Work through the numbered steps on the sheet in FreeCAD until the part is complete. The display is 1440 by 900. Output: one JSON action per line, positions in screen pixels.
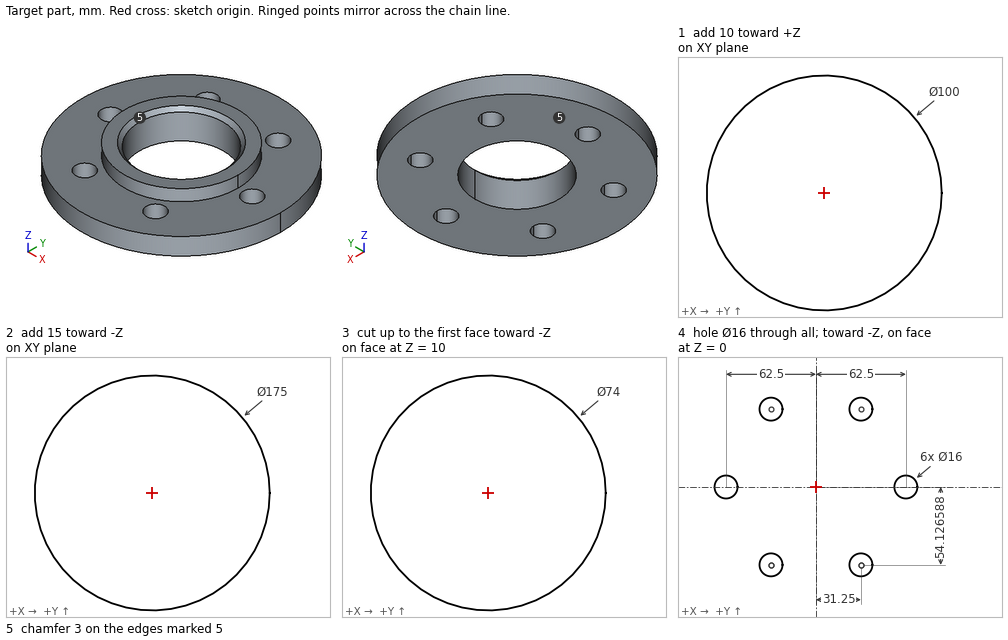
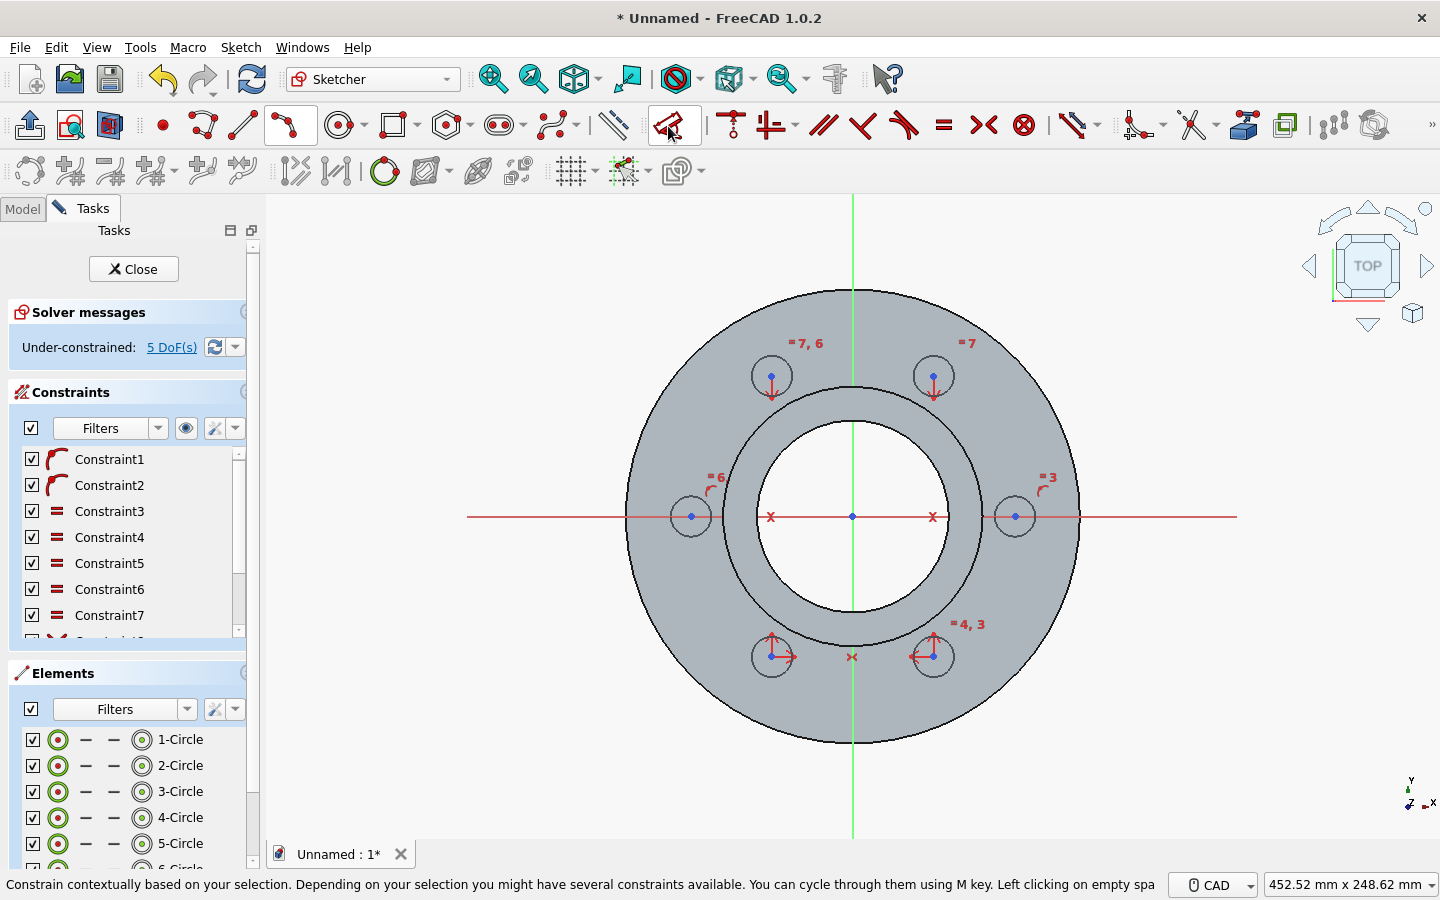
{"action": "left_click", "coordinate": [1029, 502]}
{"action": "left_click", "coordinate": [1051, 479]}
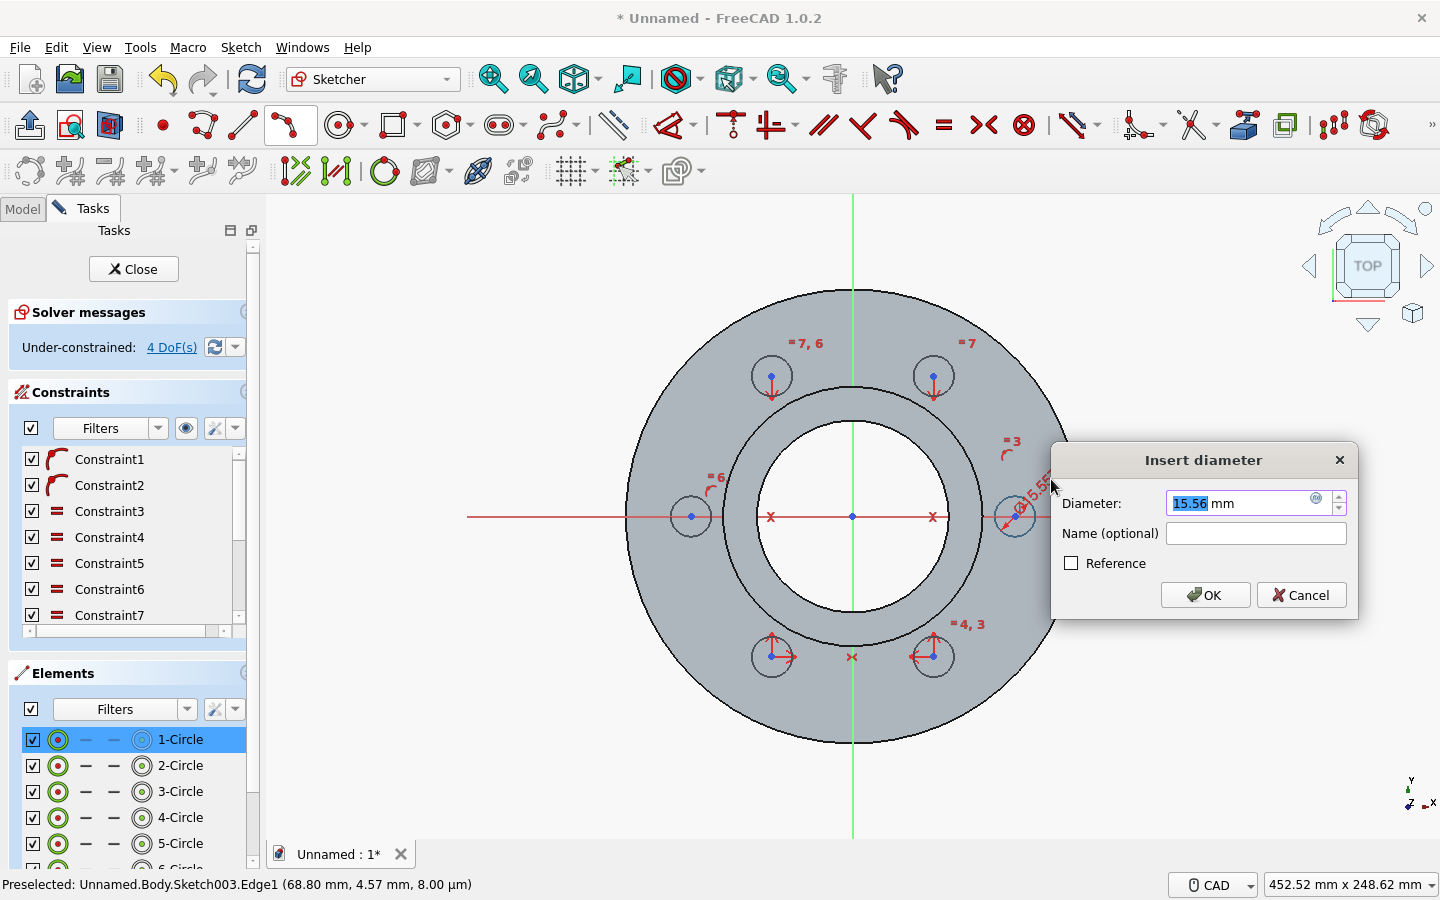
{"action": "type", "text": "16"}
{"action": "key", "text": "Return"}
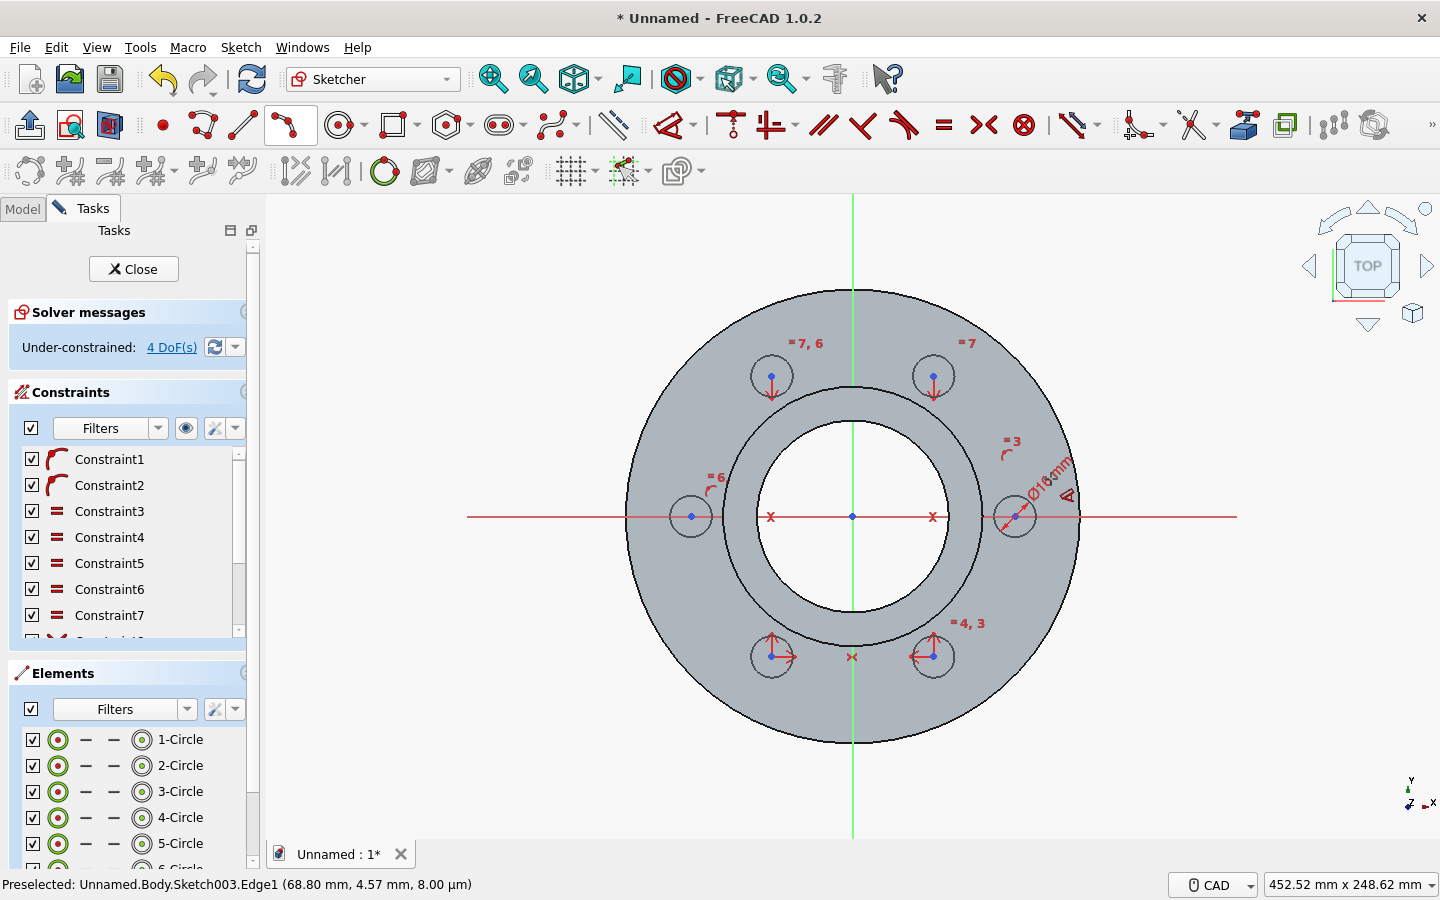
{"action": "left_click", "coordinate": [1015, 516]}
{"action": "left_click", "coordinate": [934, 550]}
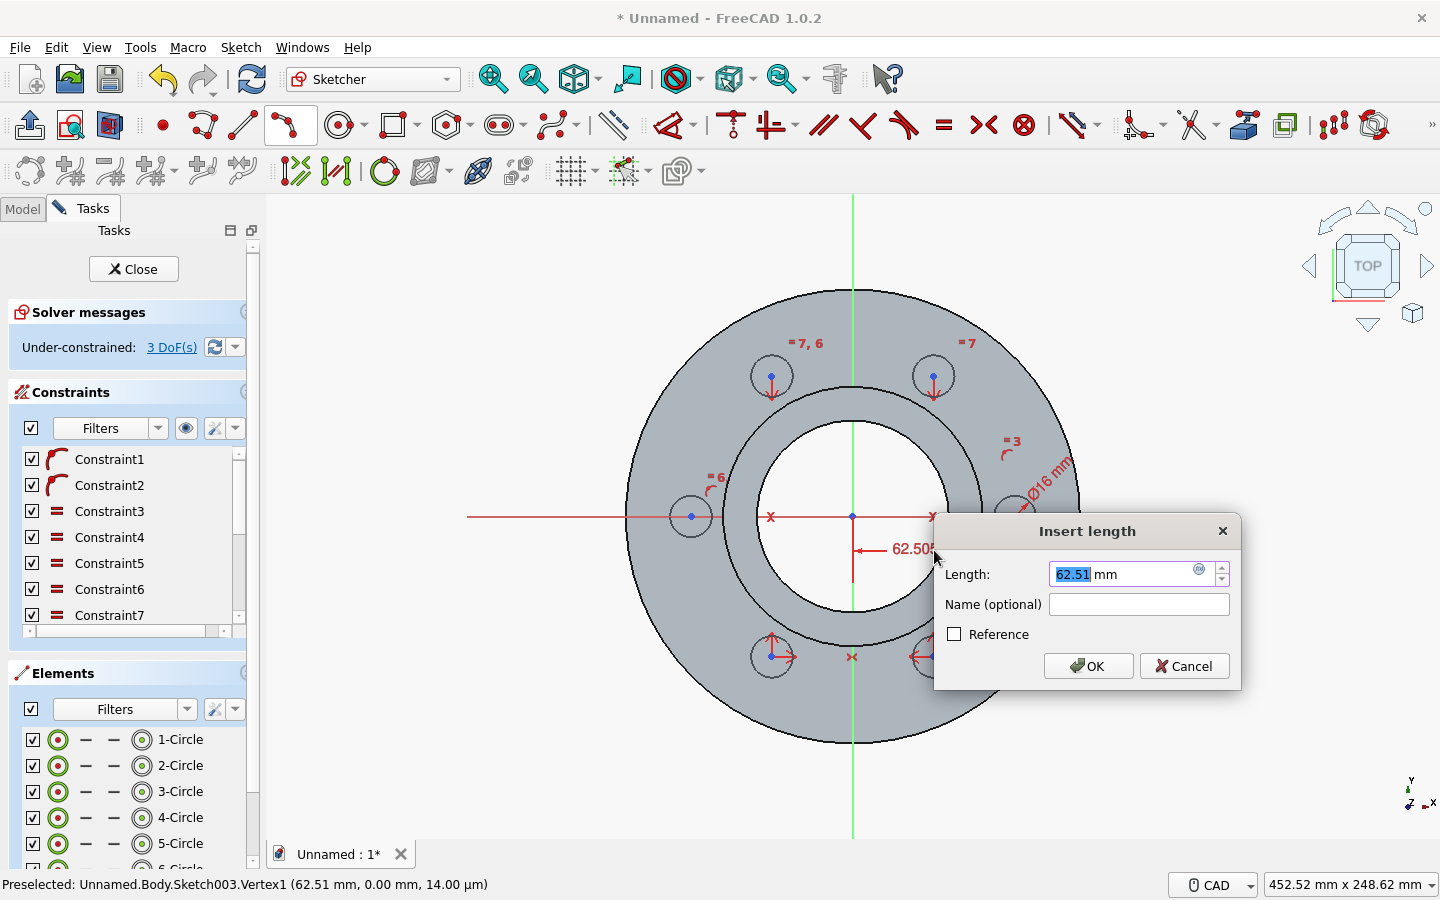
{"action": "type", "text": "62.5"}
{"action": "key", "text": "Return"}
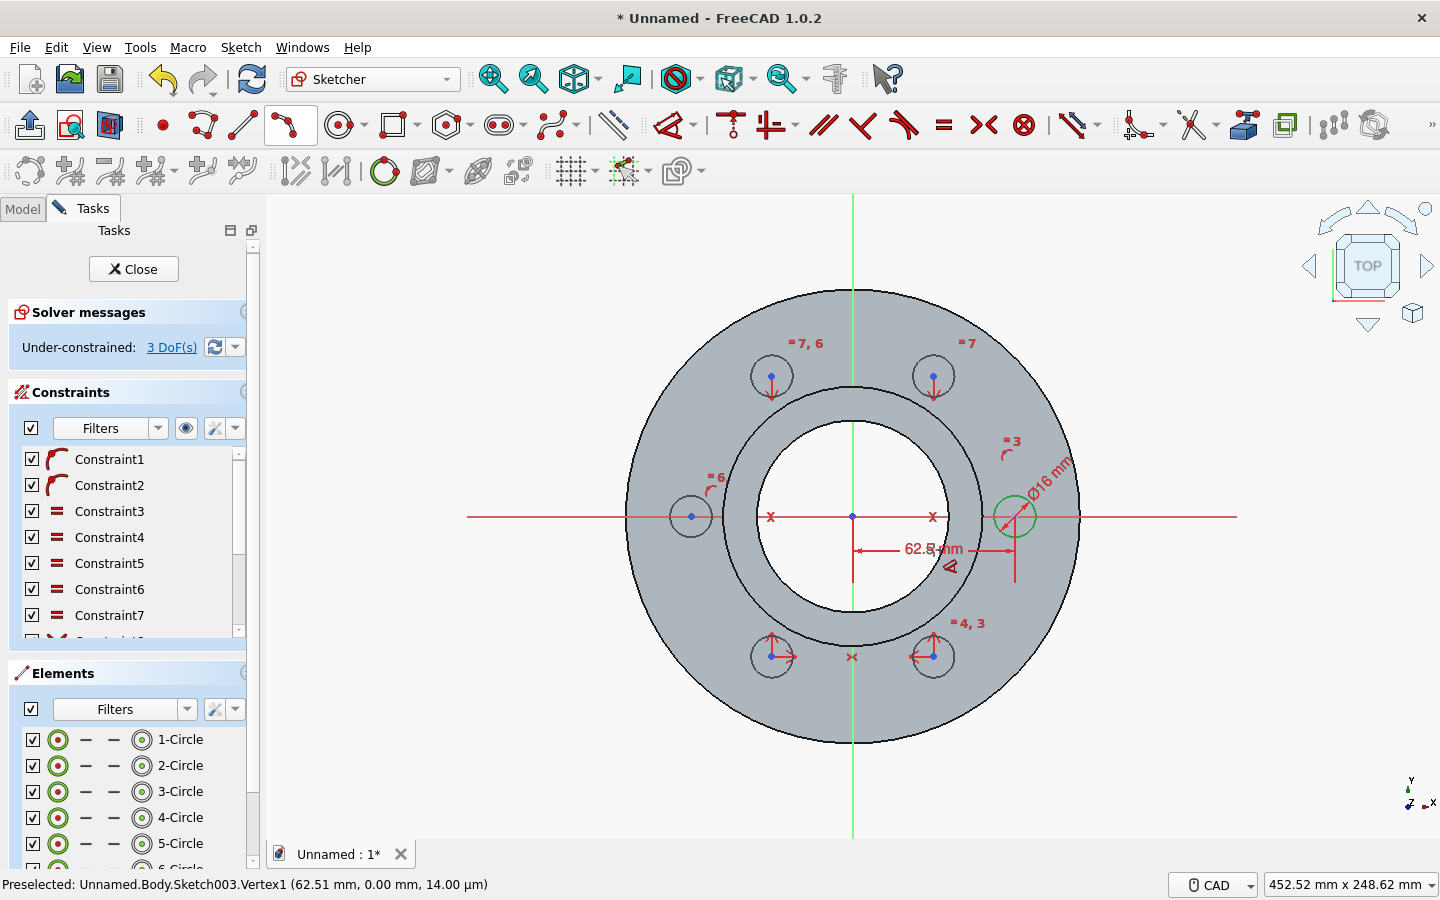
{"action": "left_click", "coordinate": [691, 516]}
{"action": "left_click", "coordinate": [772, 550]}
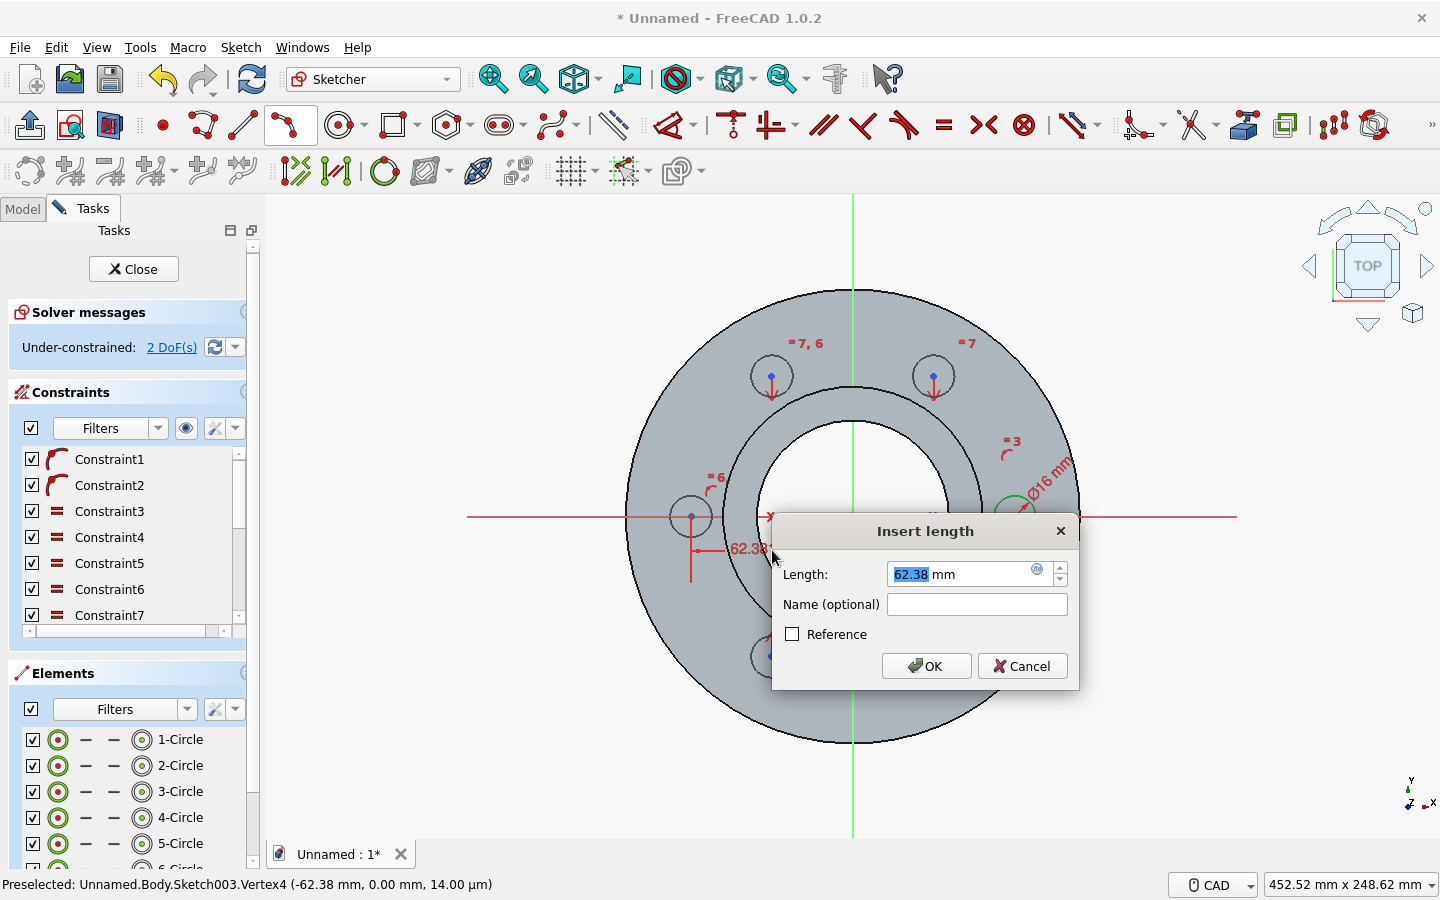
{"action": "type", "text": "62.5"}
{"action": "key", "text": "Return"}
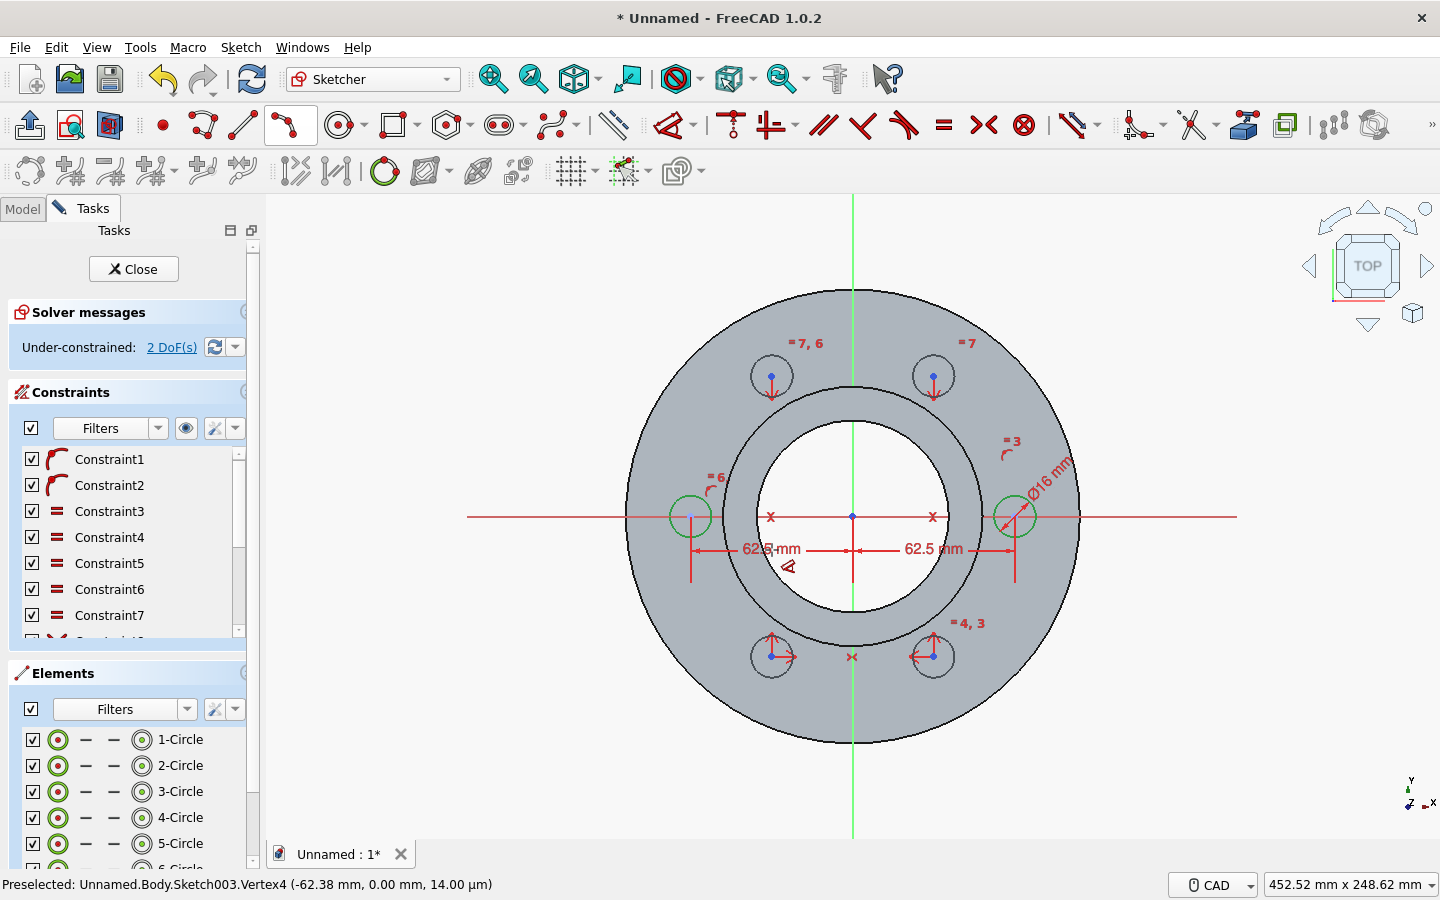
{"action": "left_click", "coordinate": [934, 657]}
{"action": "left_click", "coordinate": [893, 691]}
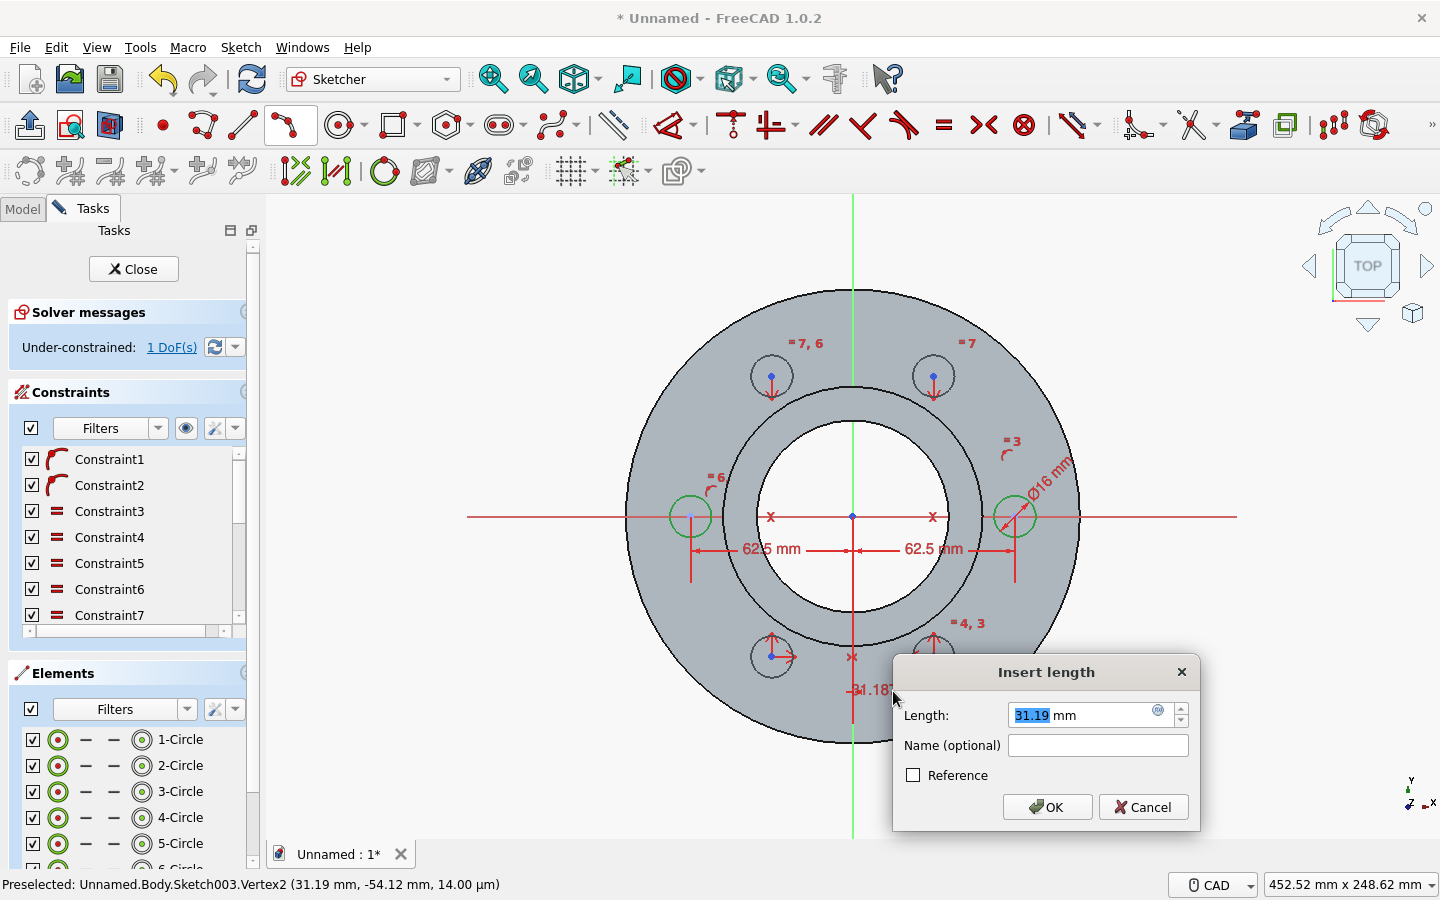
{"action": "type", "text": "31.25"}
{"action": "key", "text": "Return"}